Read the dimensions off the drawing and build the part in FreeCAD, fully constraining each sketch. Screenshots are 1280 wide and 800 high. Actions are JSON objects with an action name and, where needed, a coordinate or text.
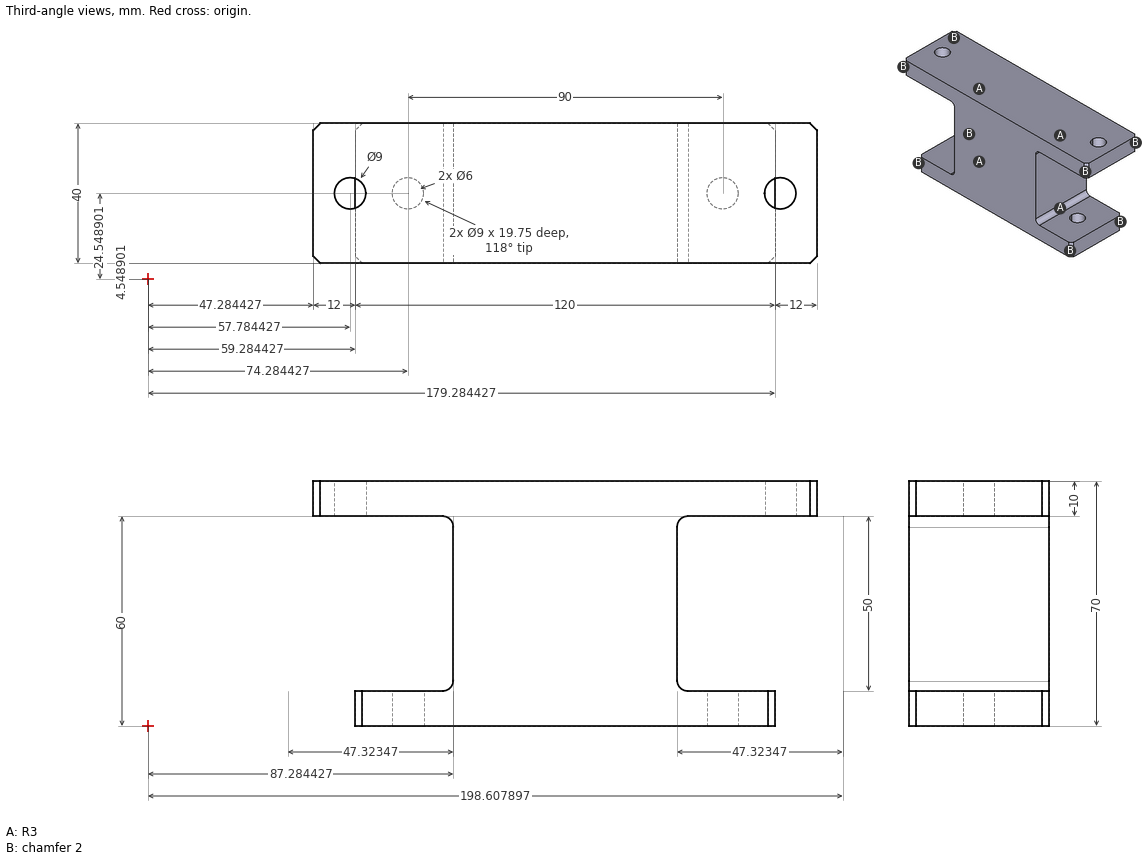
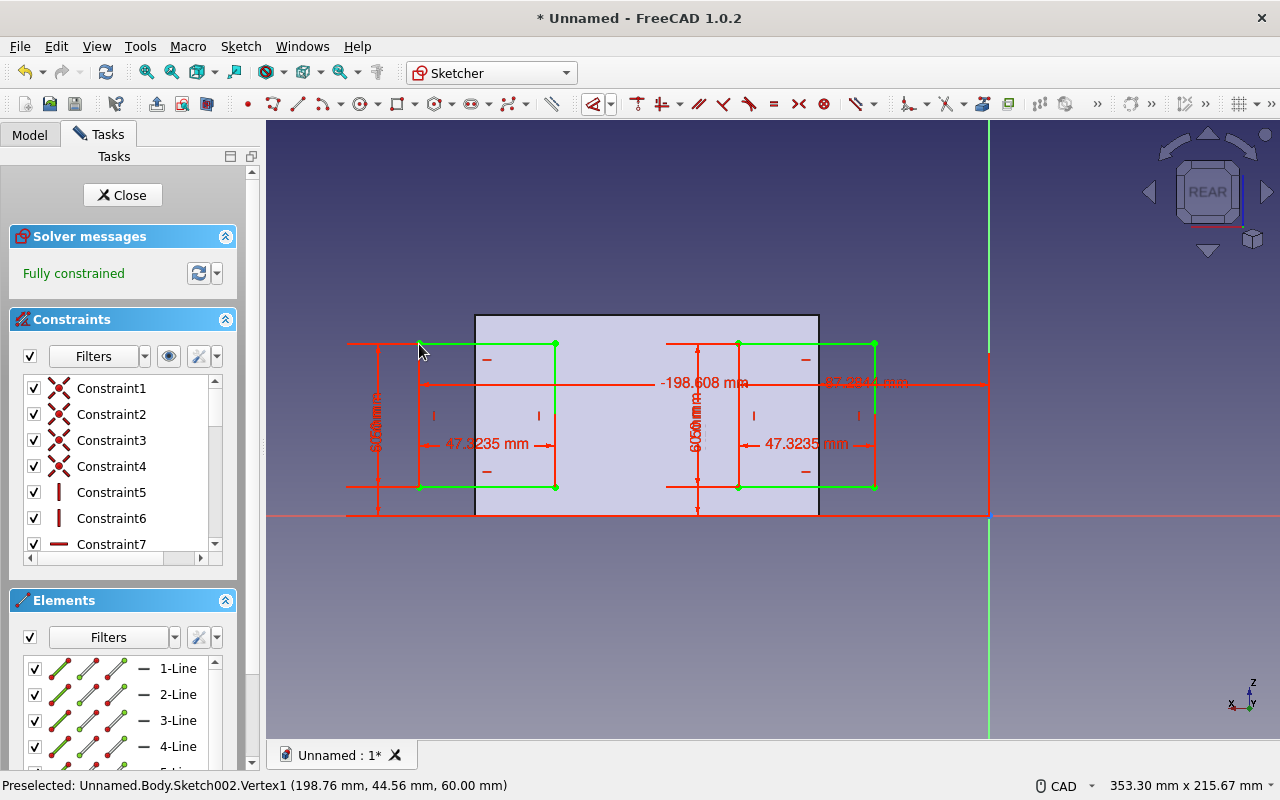
{"action": "left_click", "coordinate": [123, 195]}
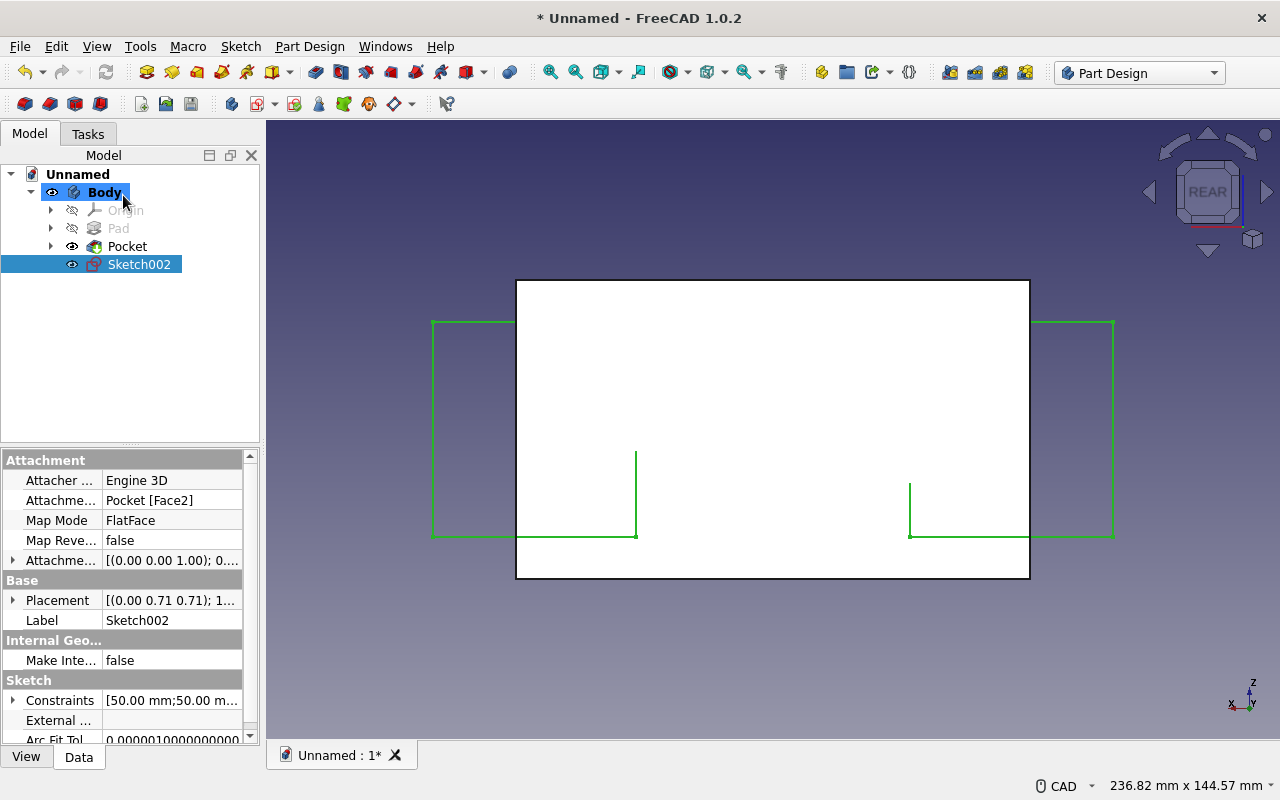
{"action": "left_click", "coordinate": [316, 72]}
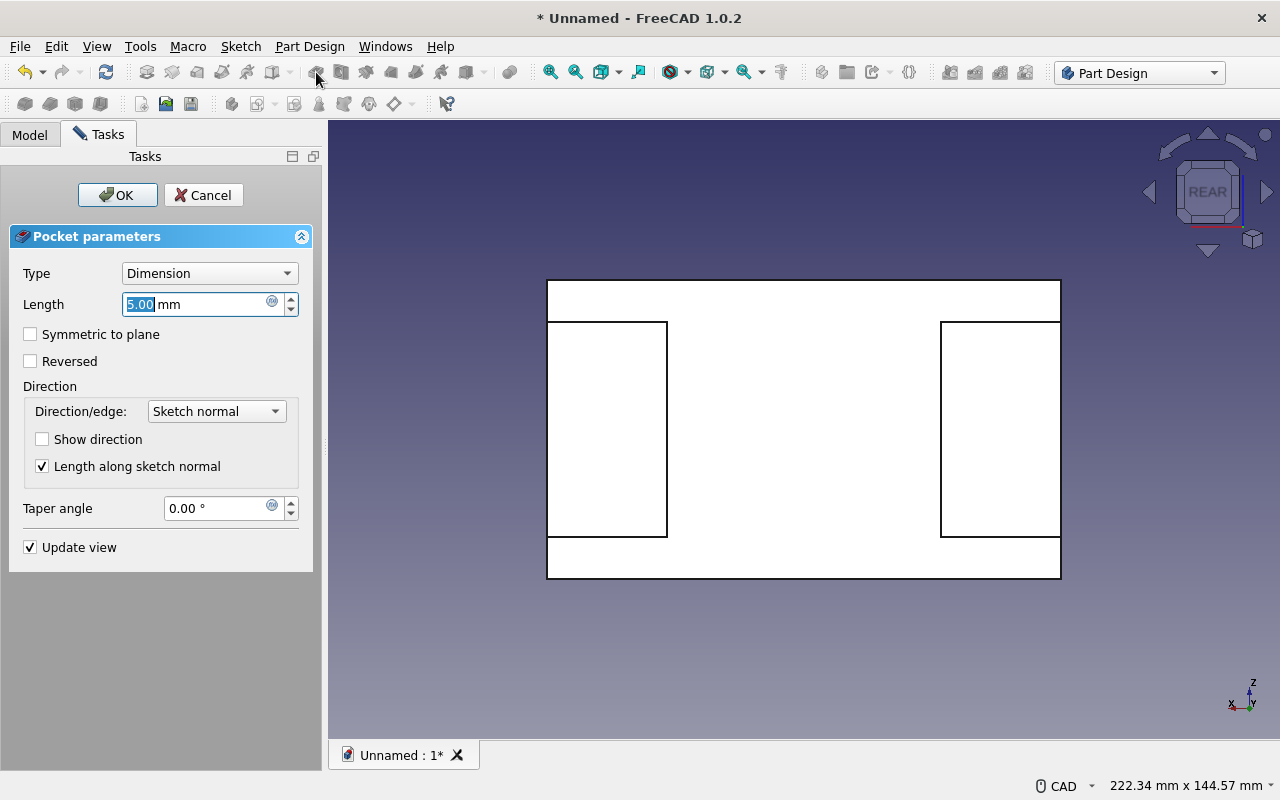
{"action": "left_click", "coordinate": [210, 274]}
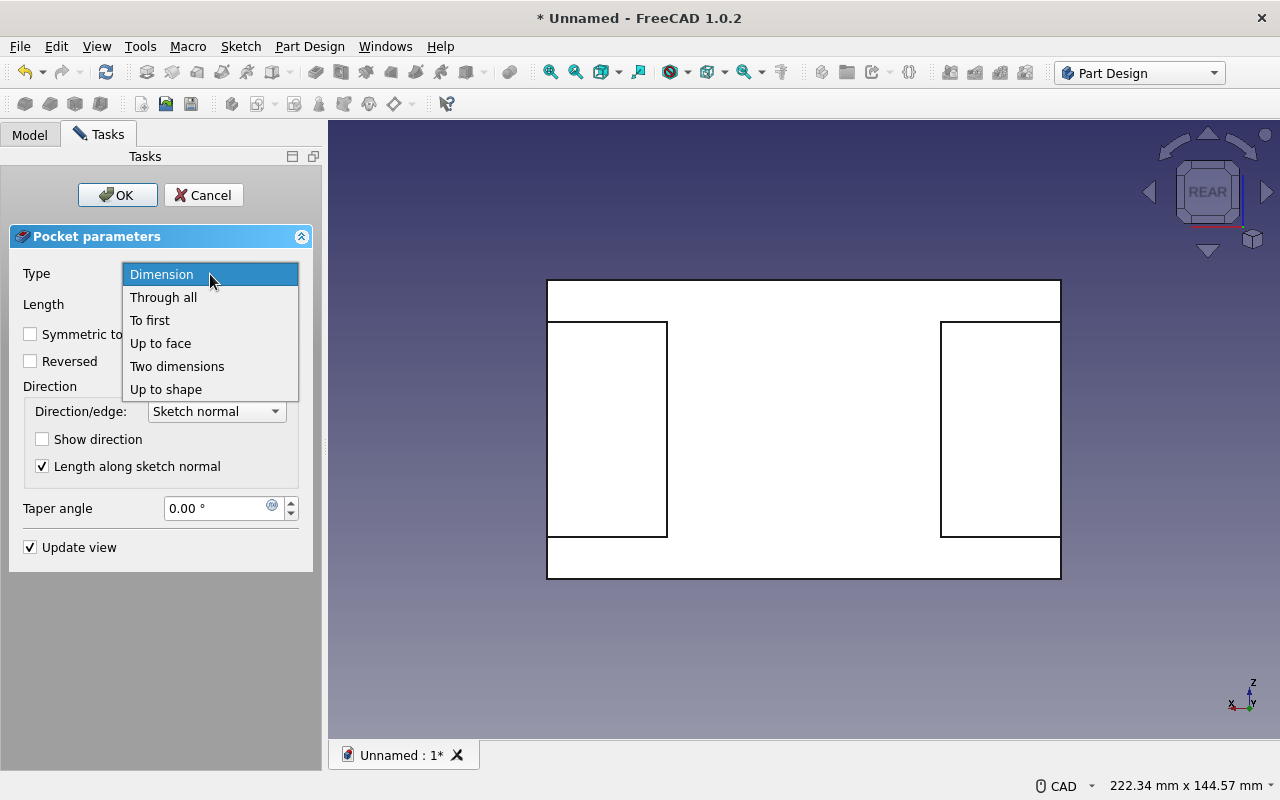
{"action": "left_click", "coordinate": [208, 298]}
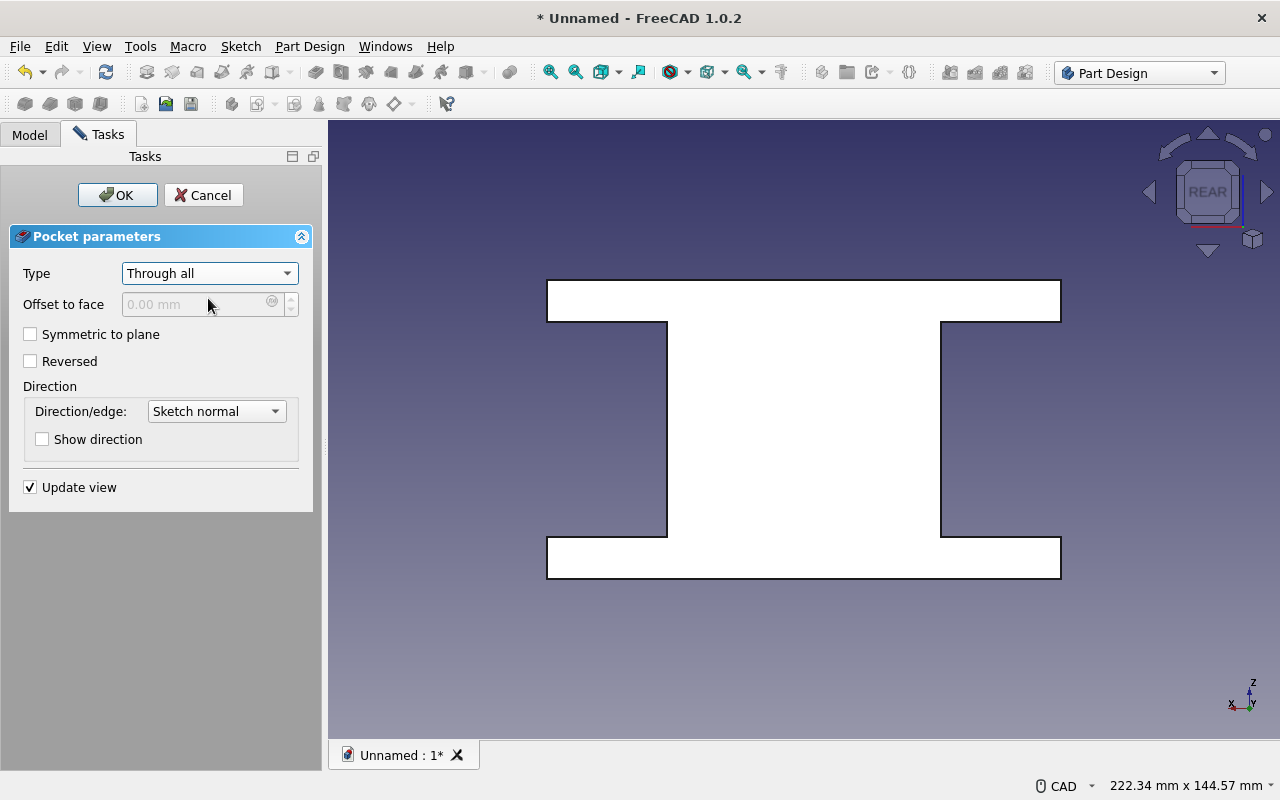
{"action": "left_click", "coordinate": [118, 195]}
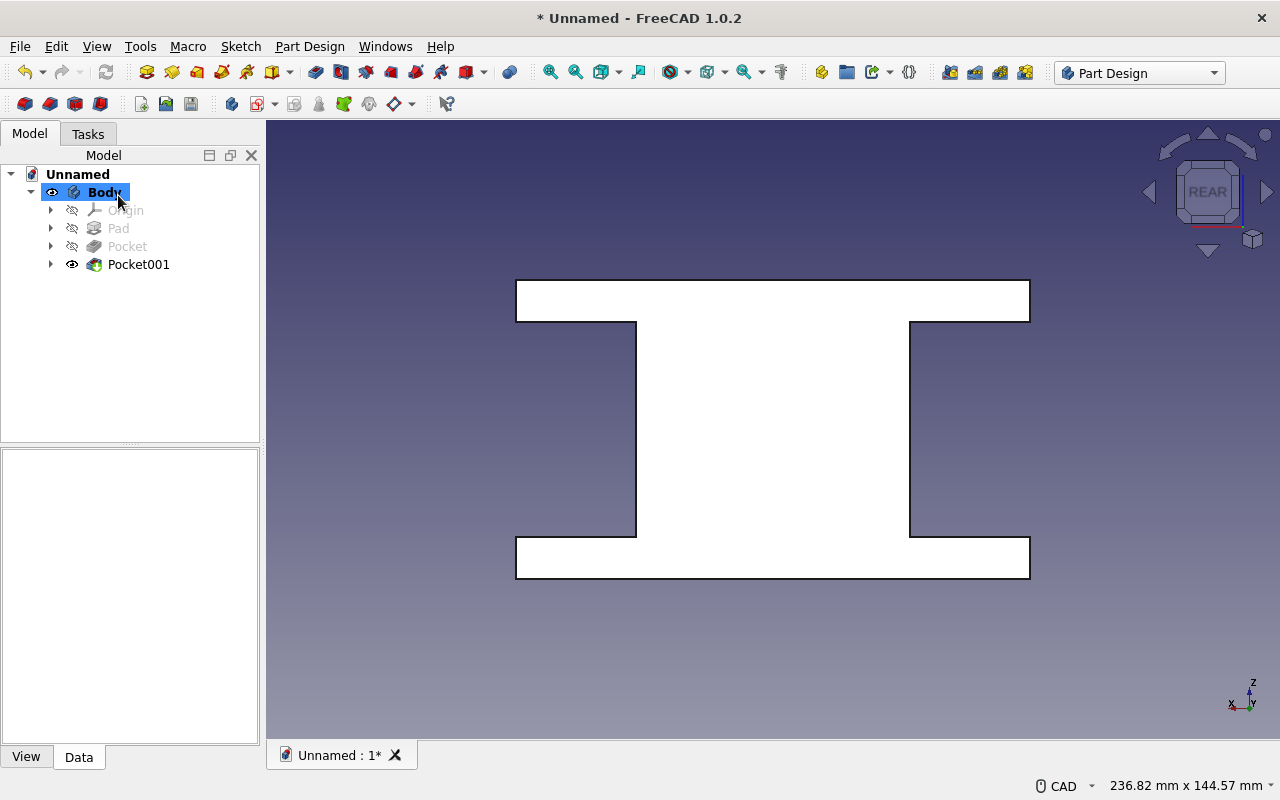
{"action": "key", "text": "0"}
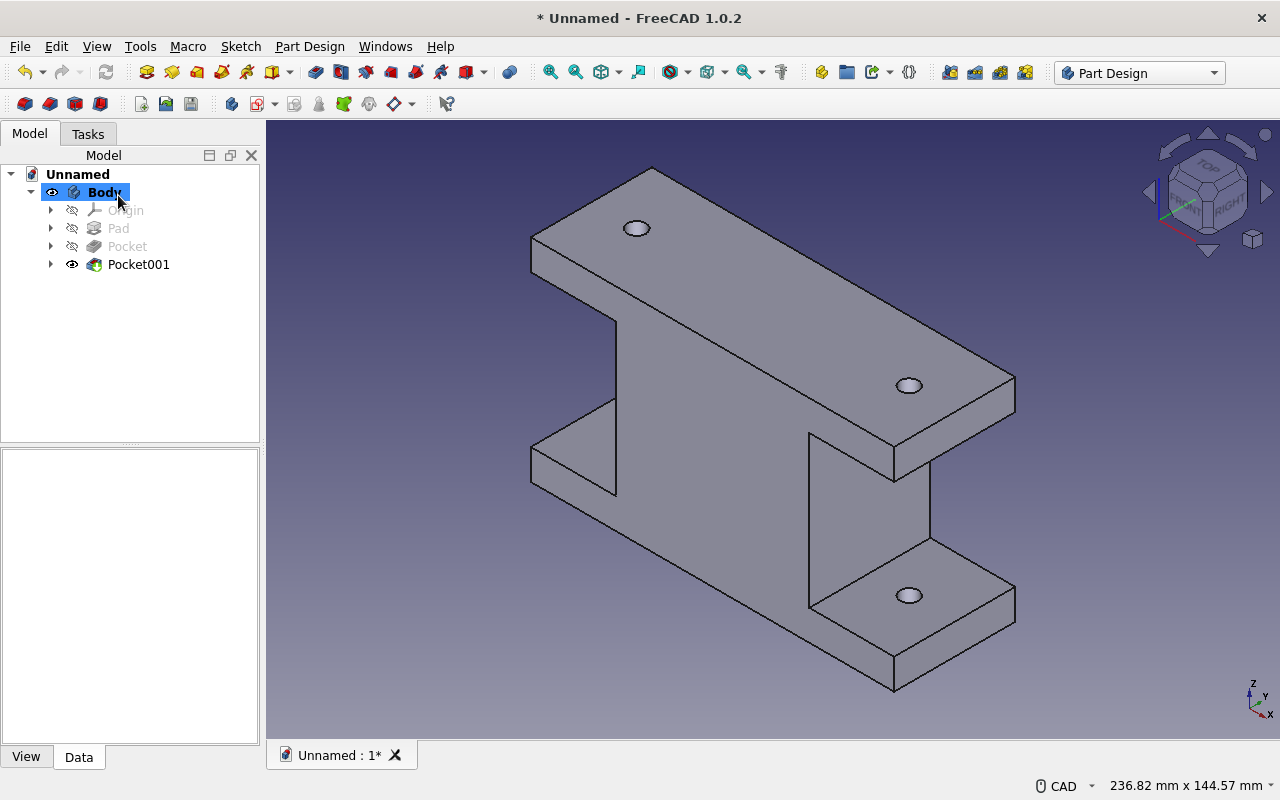
{"action": "key", "text": "2"}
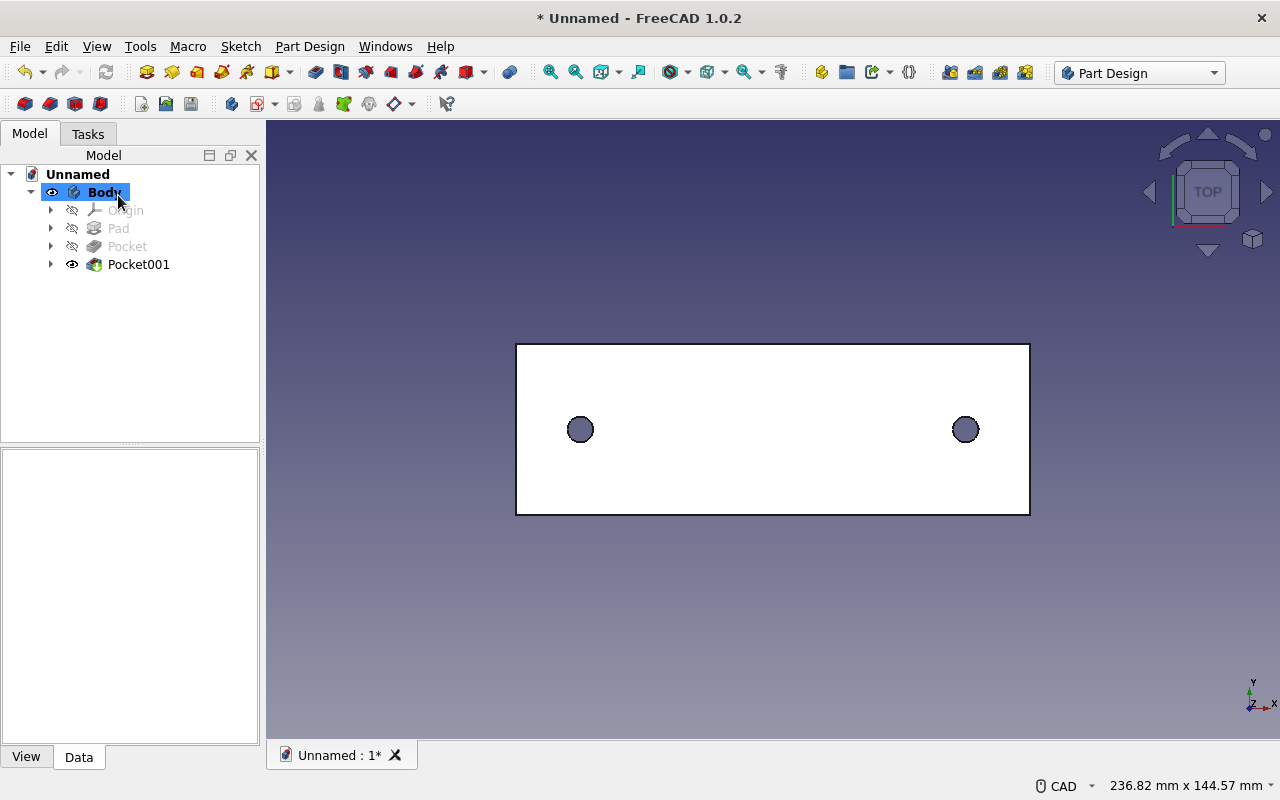
{"action": "key", "text": "1"}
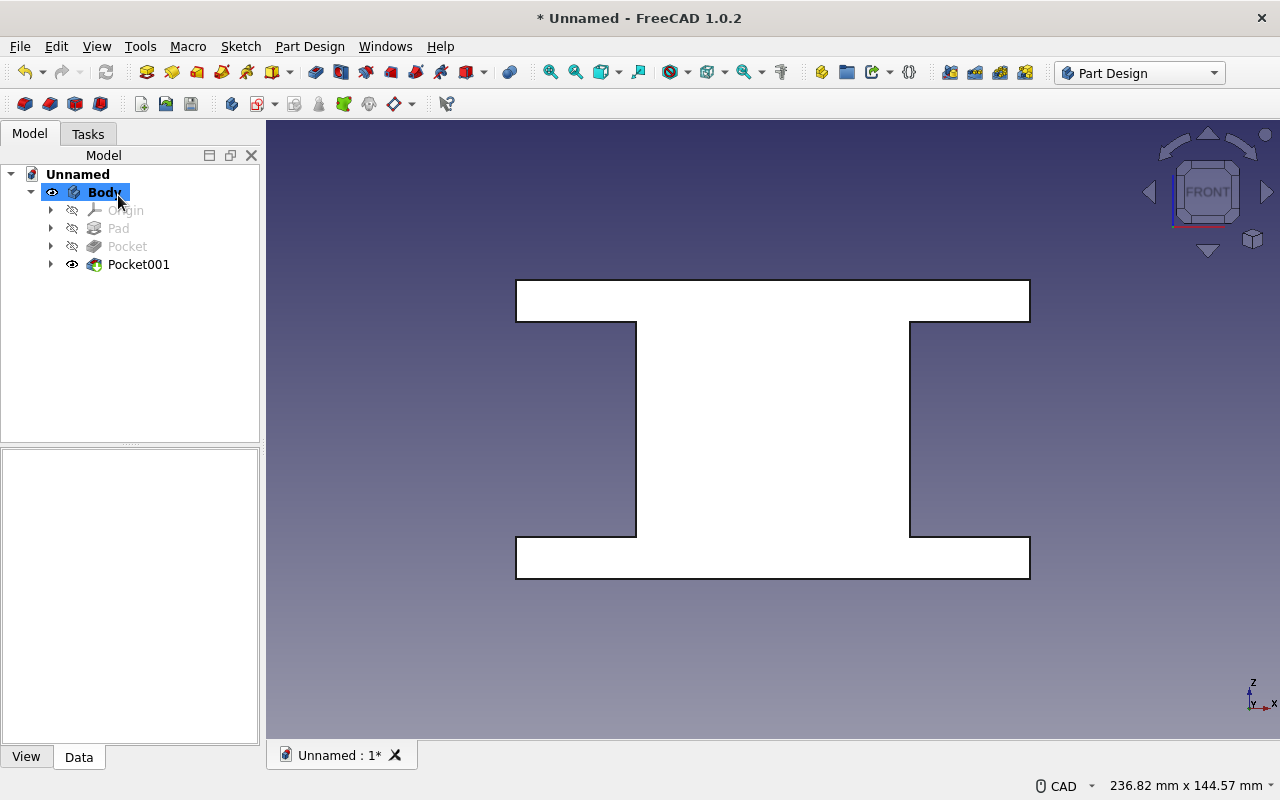
{"action": "key", "text": "3"}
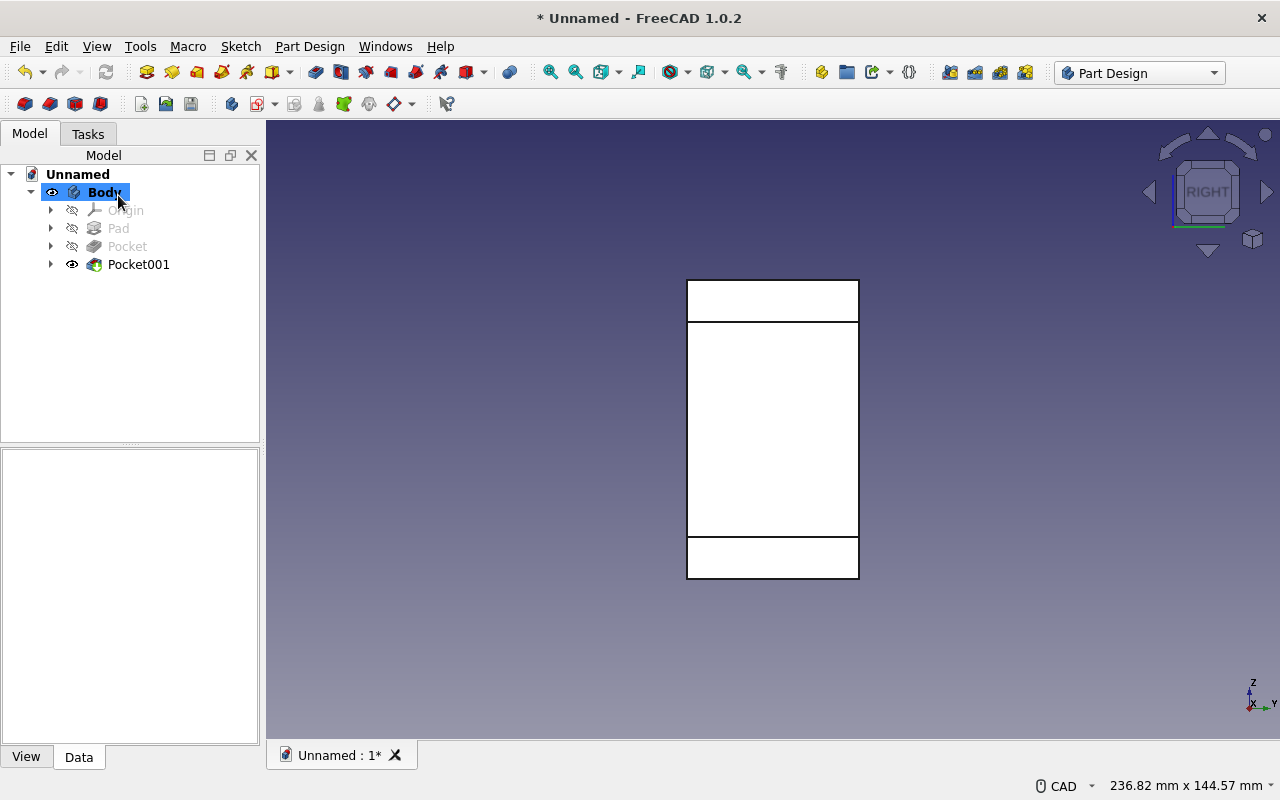
{"action": "key", "text": "5"}